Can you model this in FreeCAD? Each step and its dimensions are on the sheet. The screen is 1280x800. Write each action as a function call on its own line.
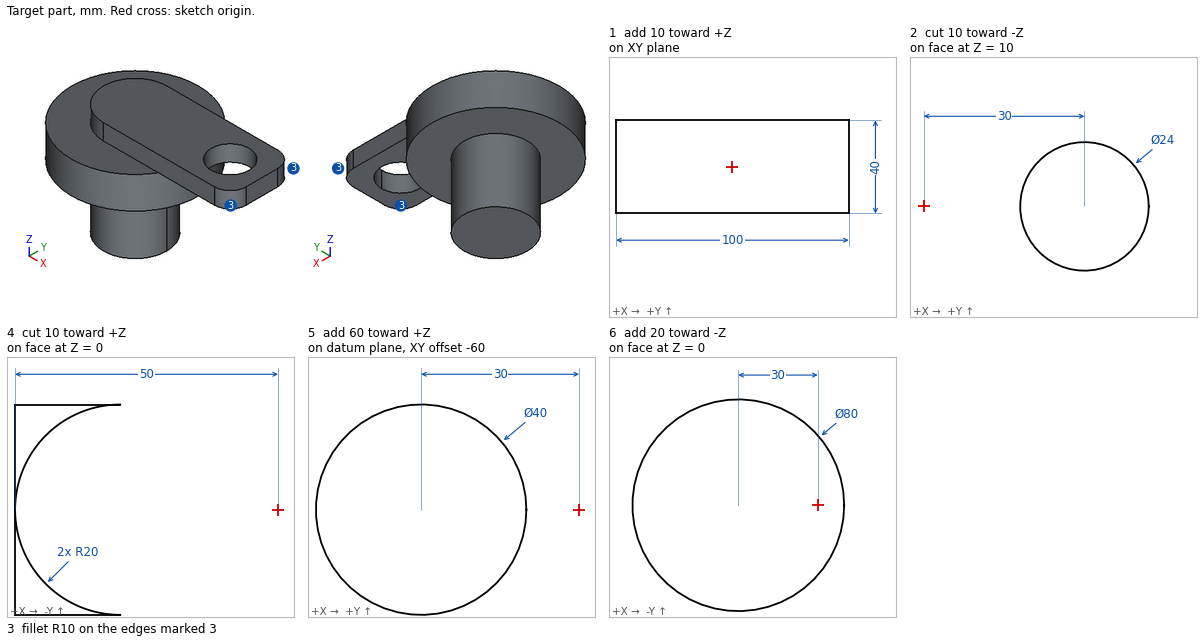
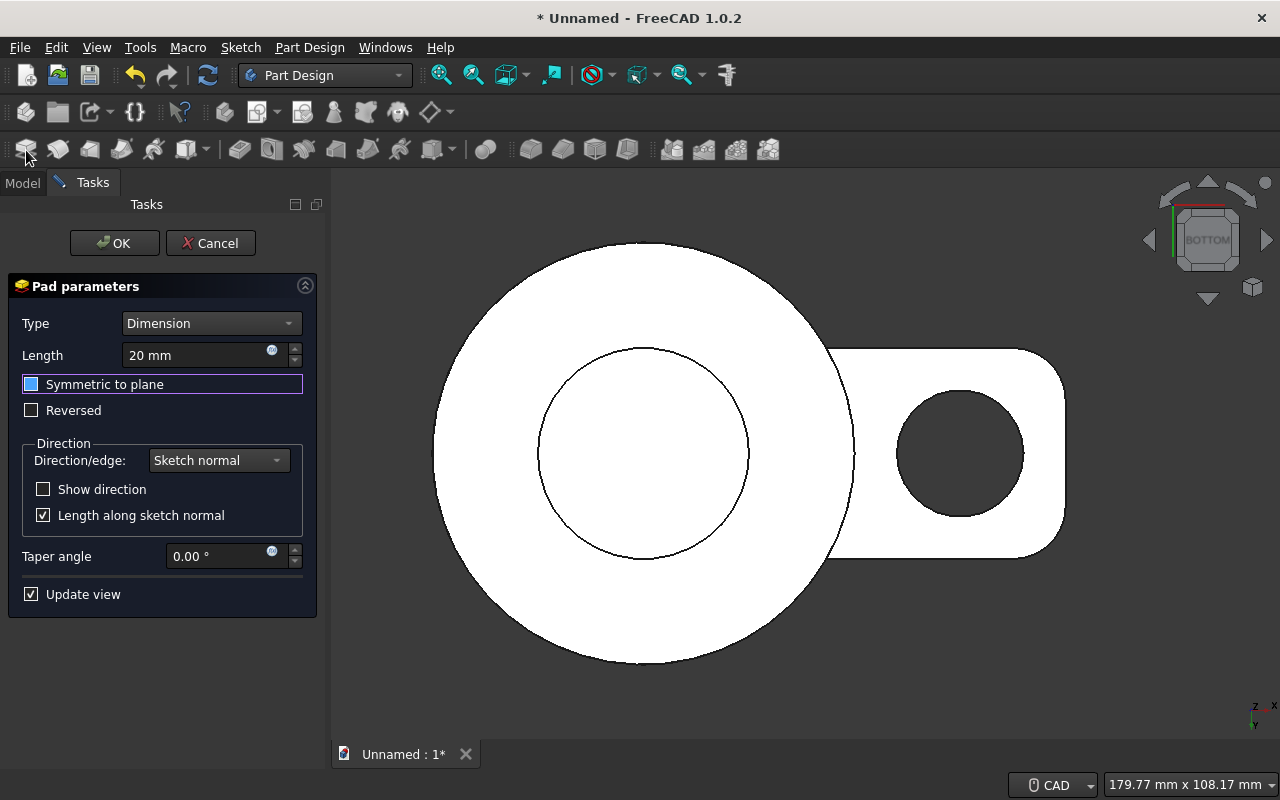
click(115, 243)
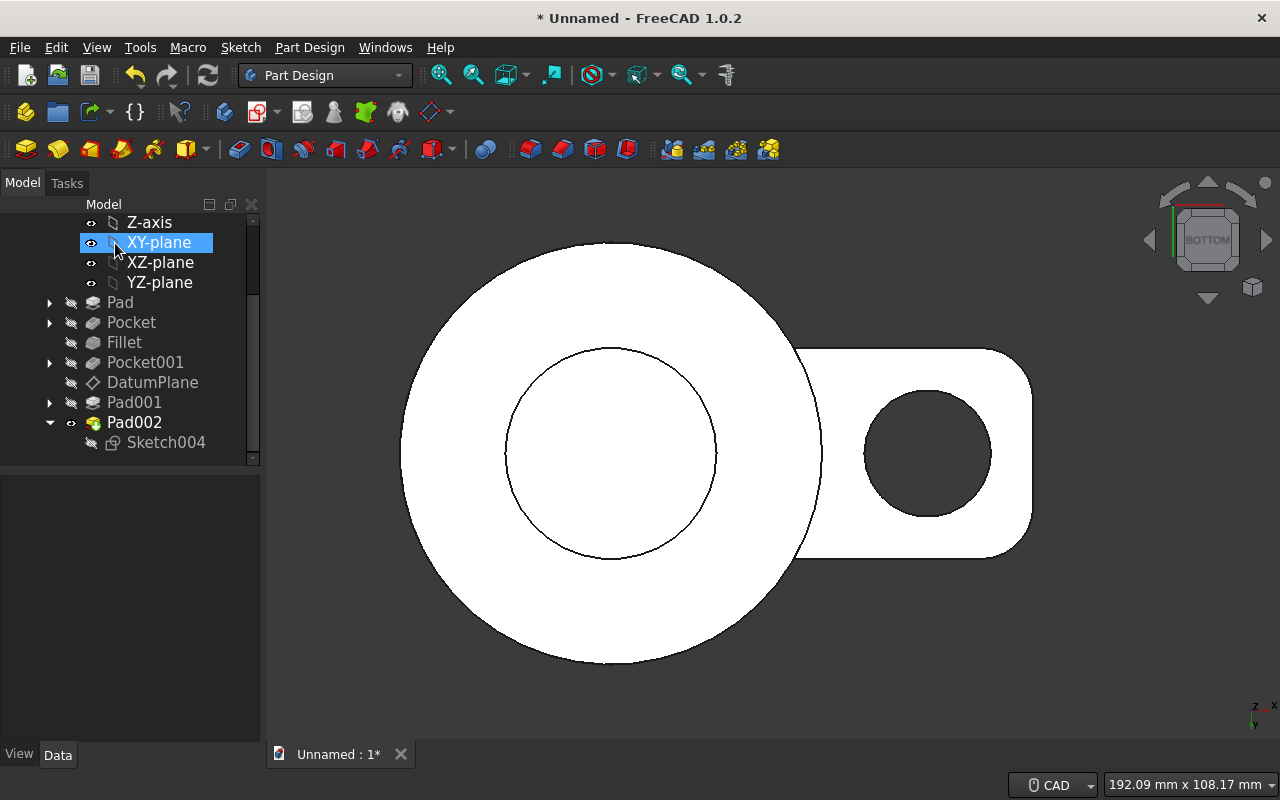
key(0)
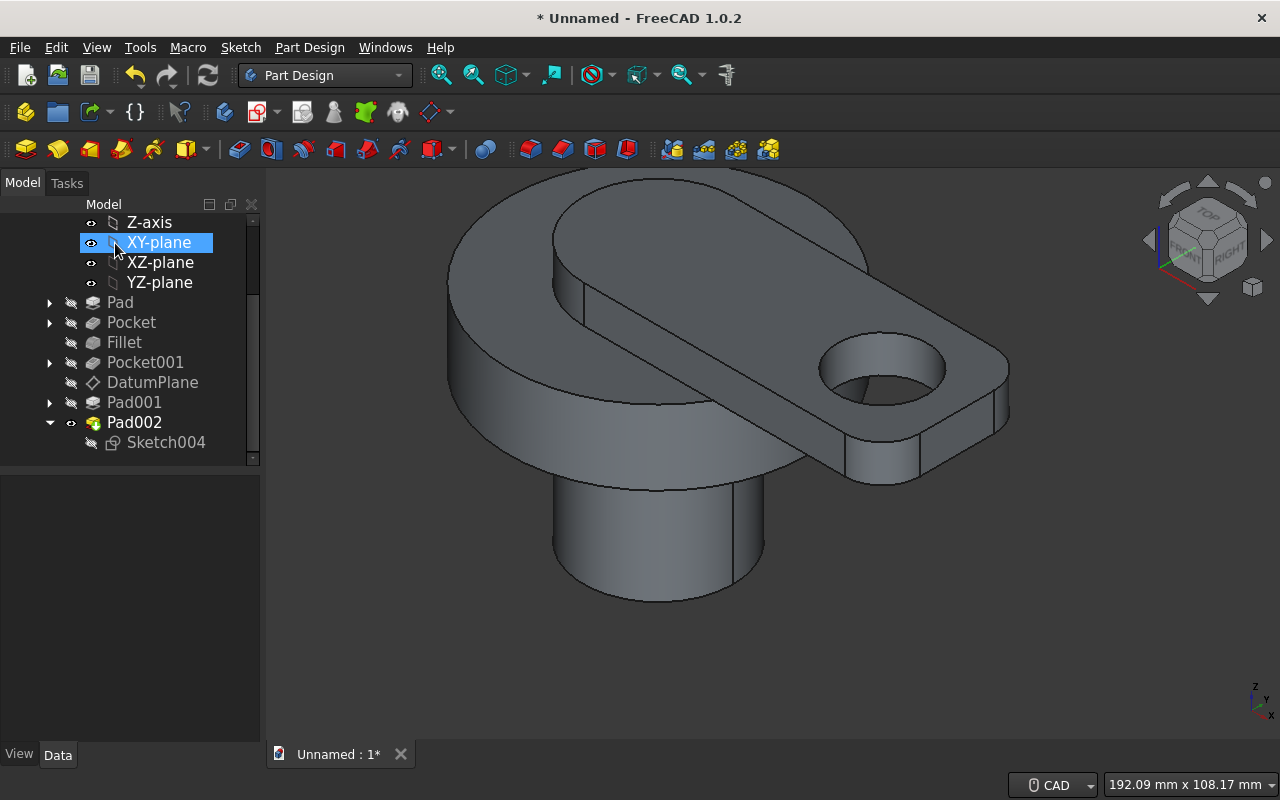
key(v)
key(f)